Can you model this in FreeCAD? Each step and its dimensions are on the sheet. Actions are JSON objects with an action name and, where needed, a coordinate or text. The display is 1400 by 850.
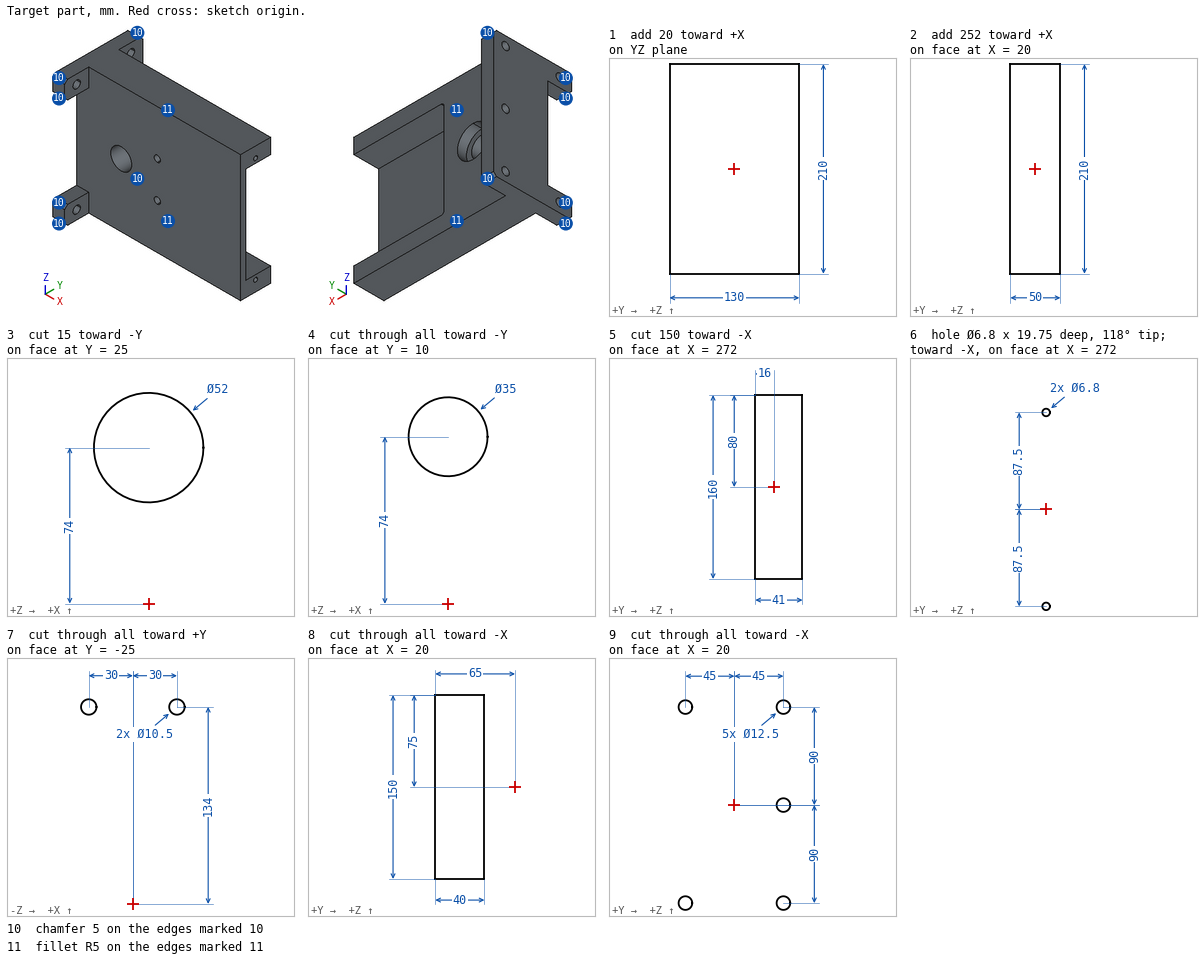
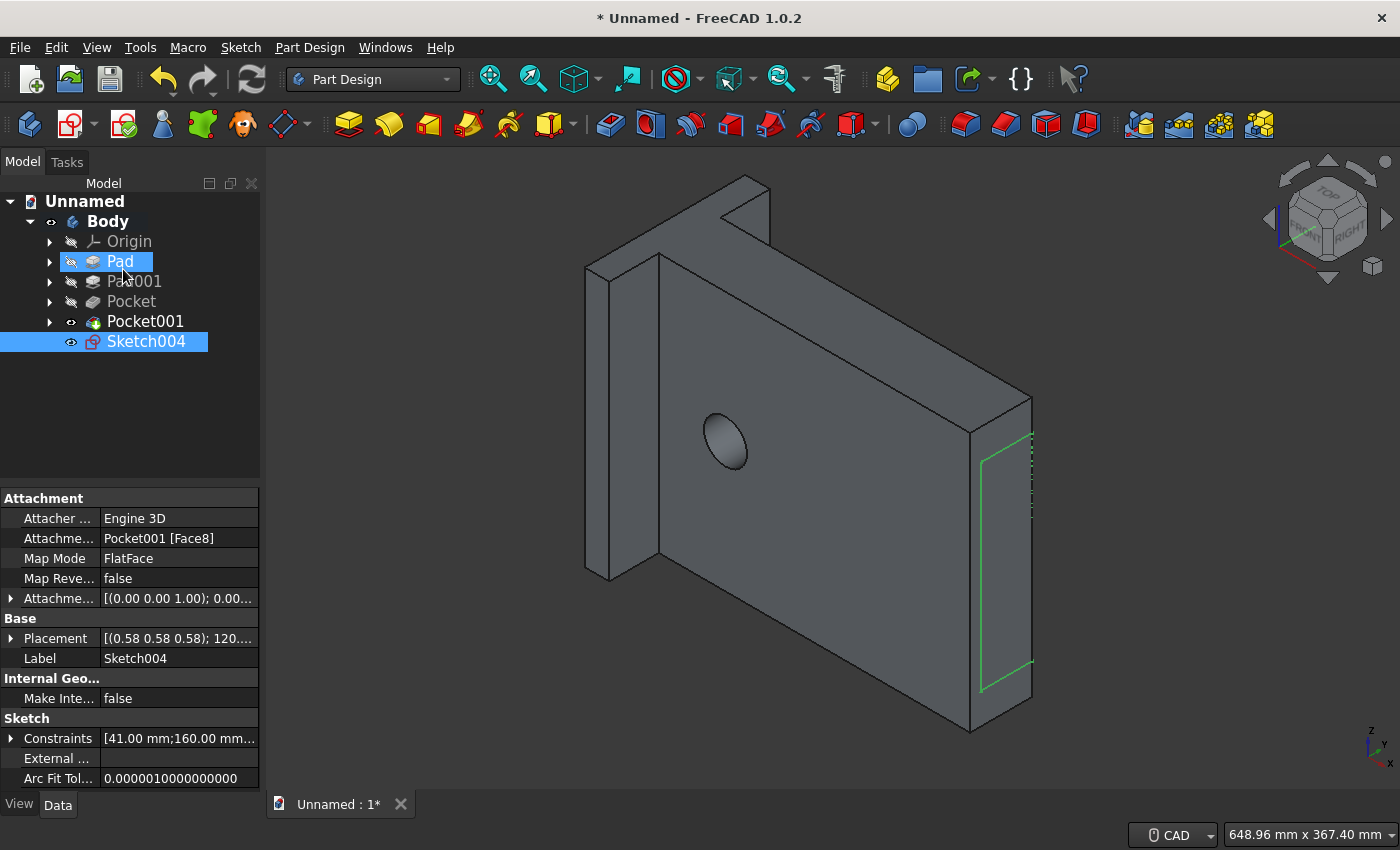
{"action": "left_click", "coordinate": [612, 124]}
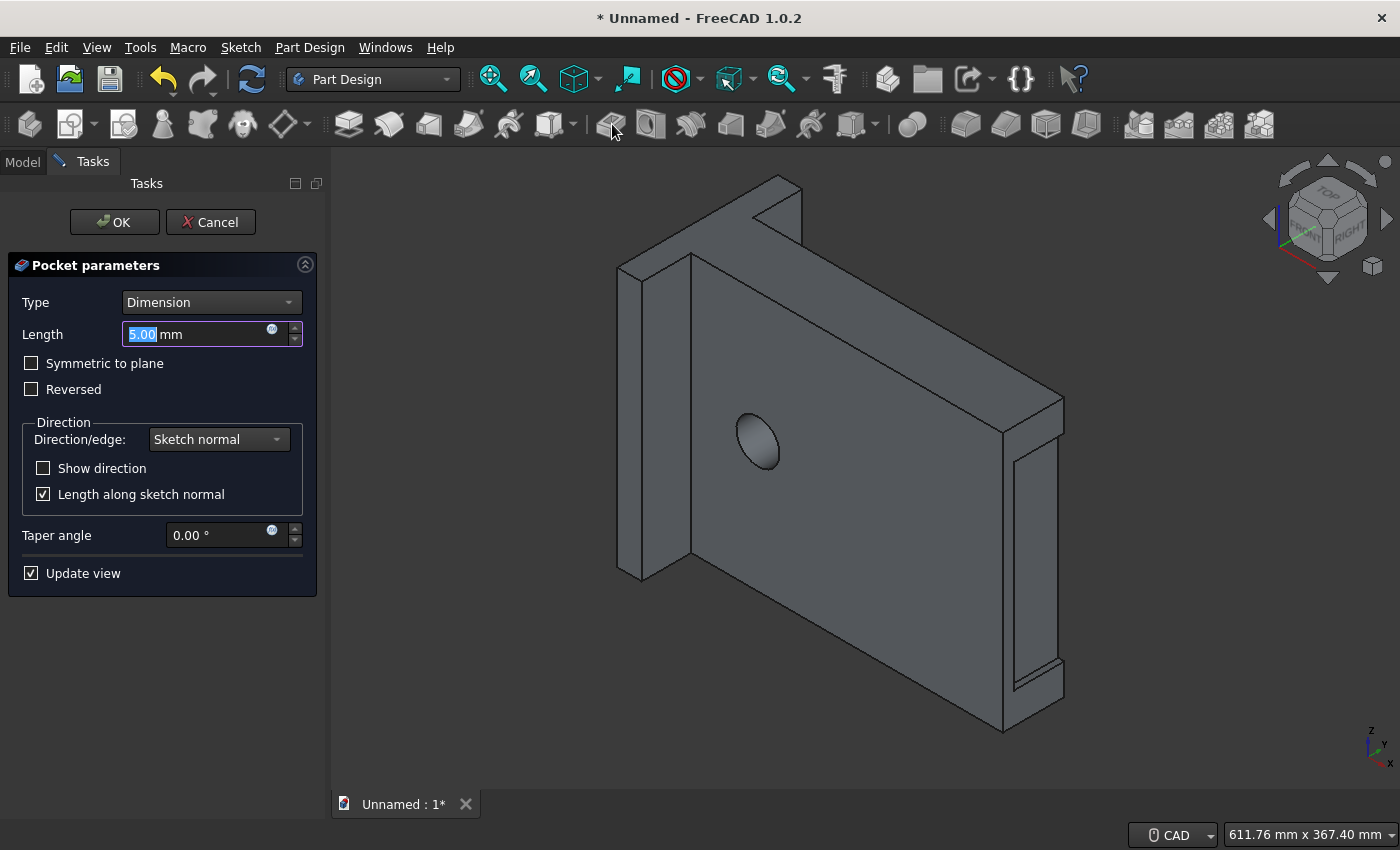
{"action": "type", "text": "150"}
{"action": "key", "text": "Tab"}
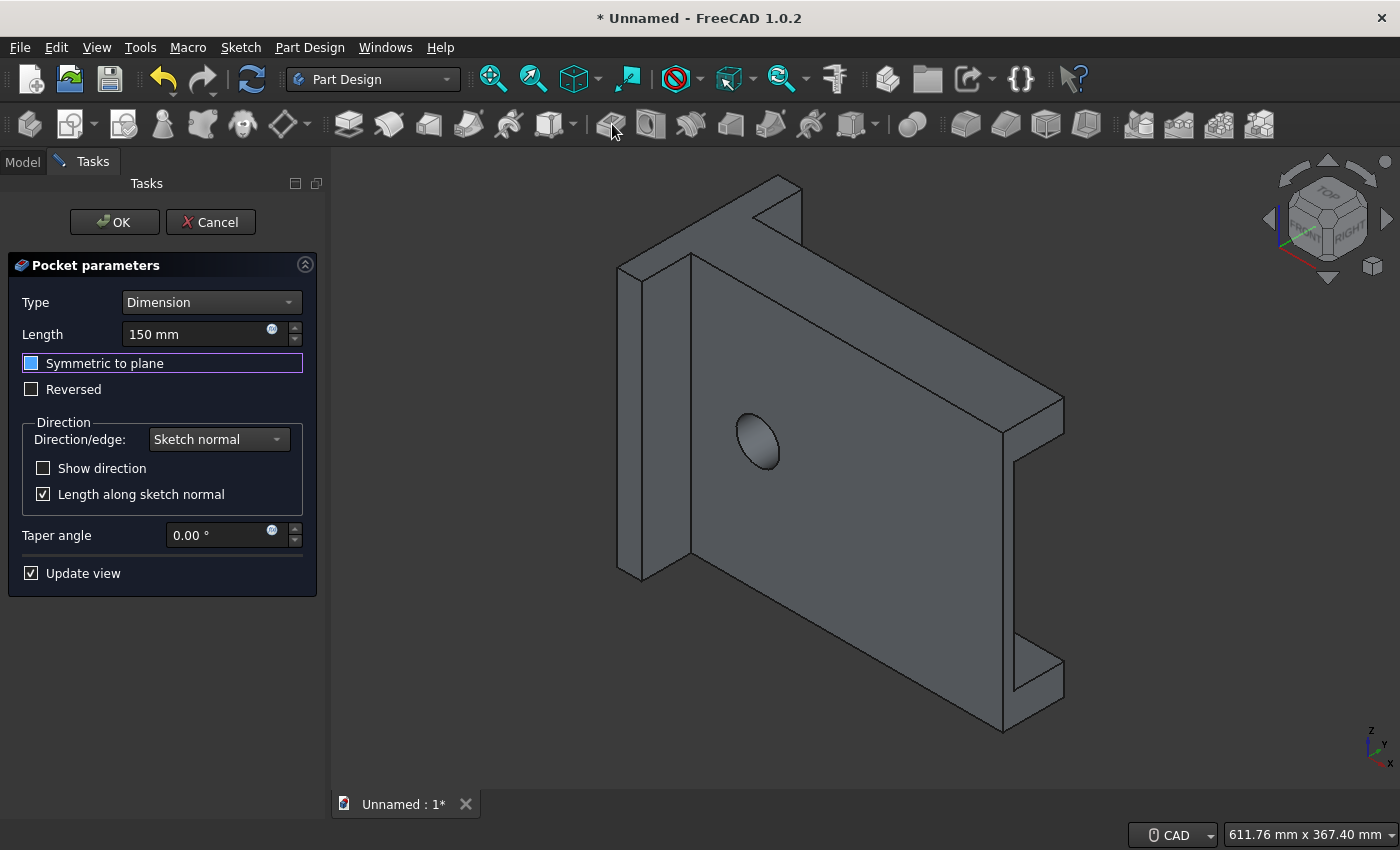
{"action": "left_click", "coordinate": [115, 222]}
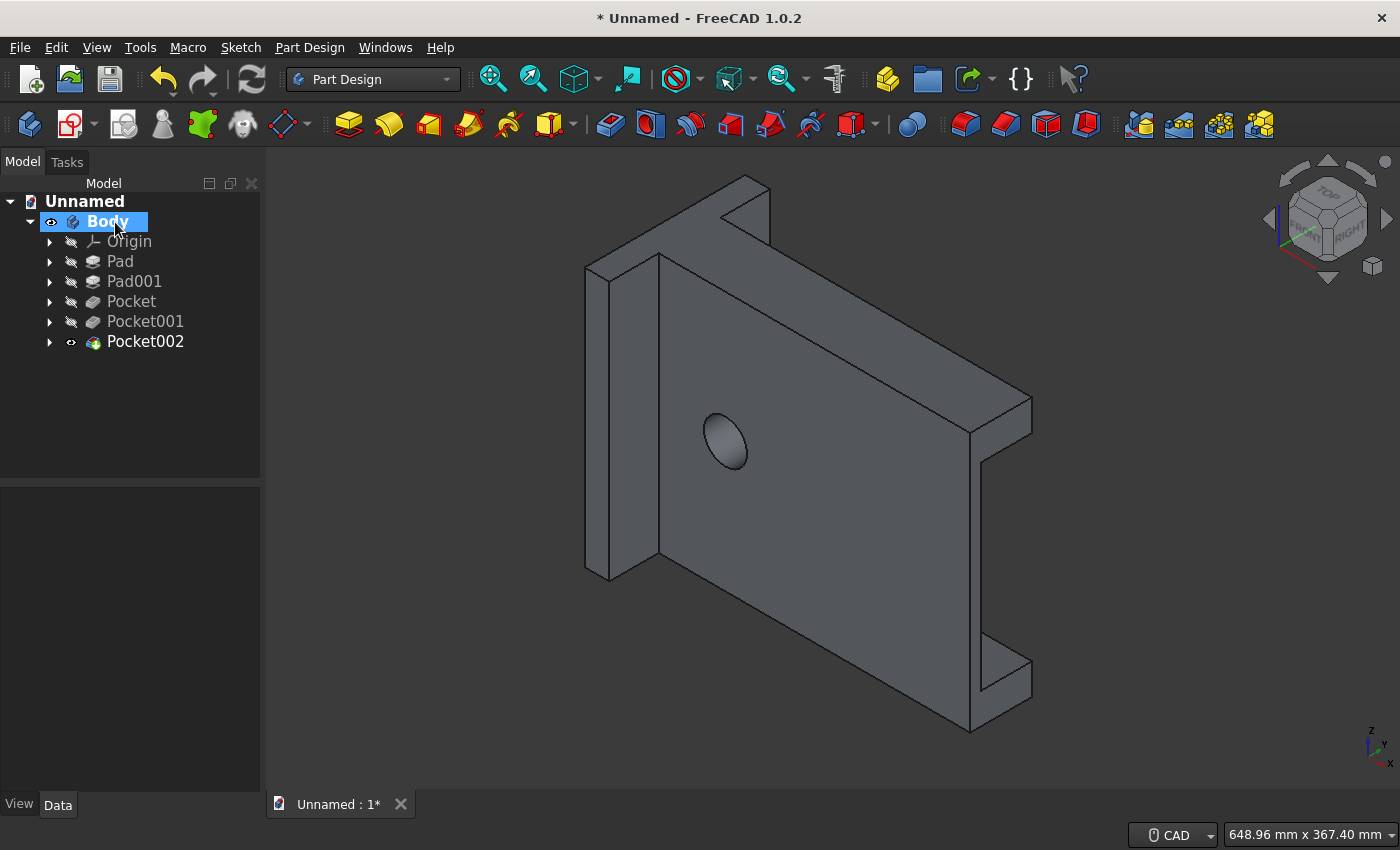
{"action": "left_click", "coordinate": [1019, 682]}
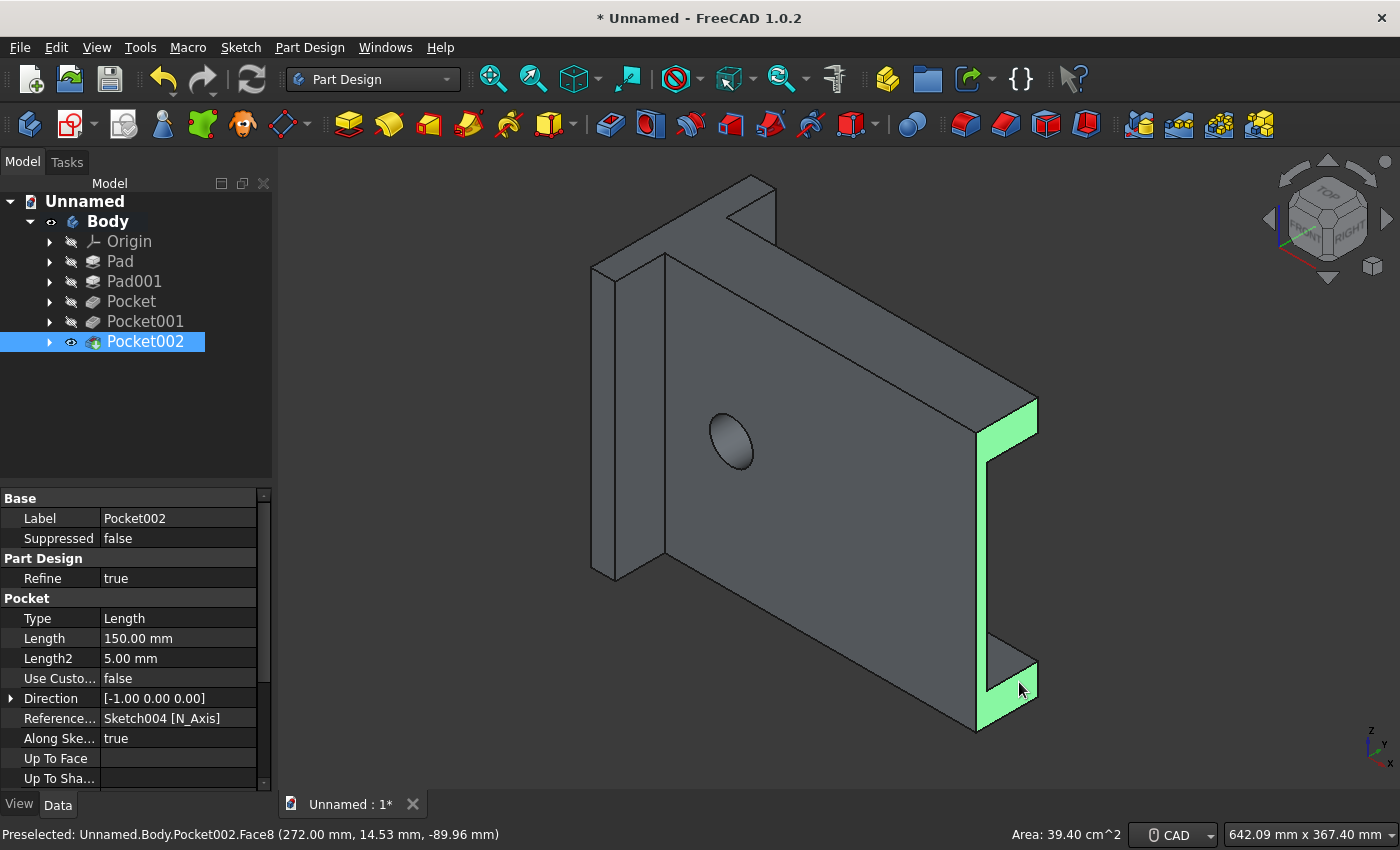
{"action": "left_click", "coordinate": [70, 124]}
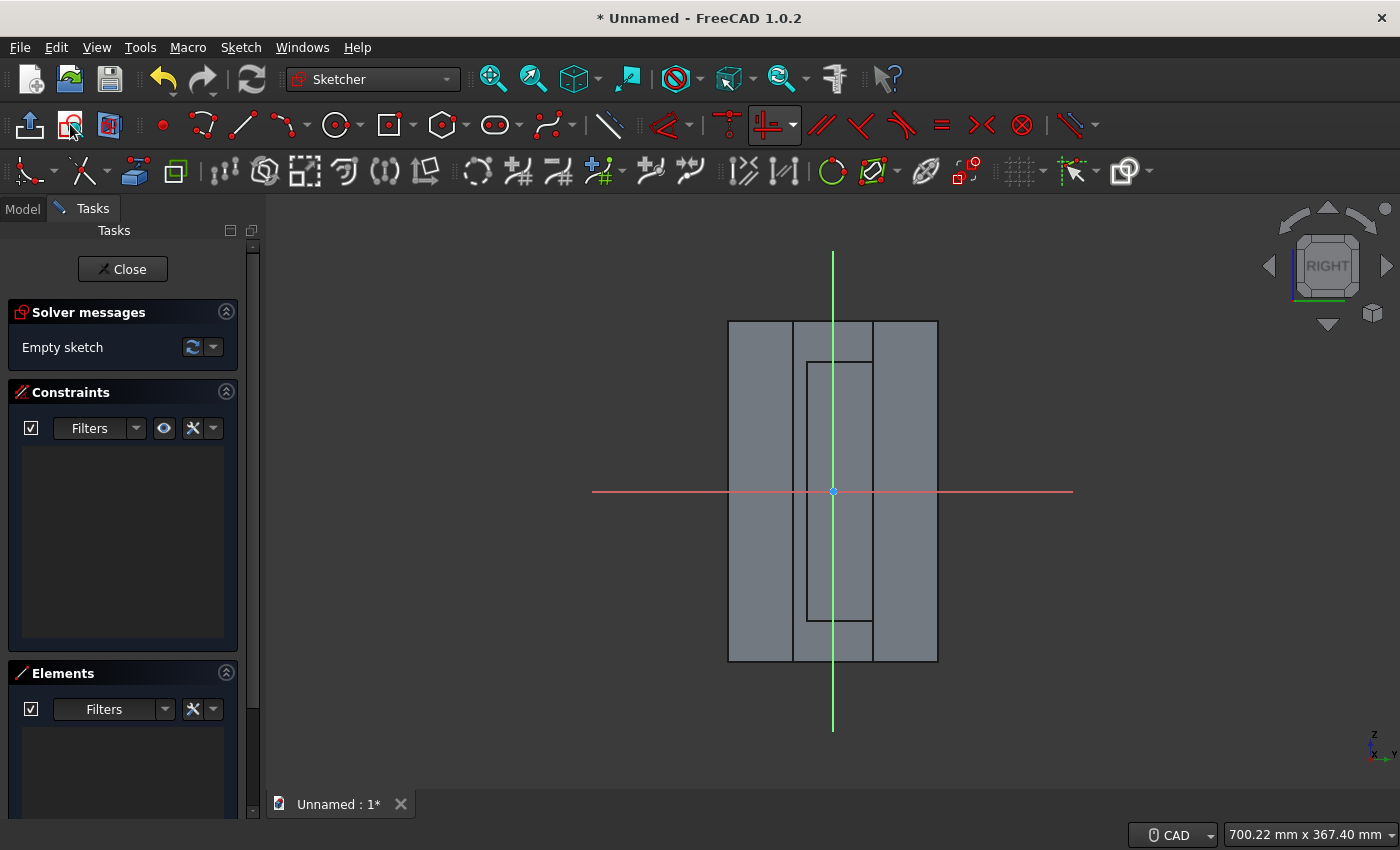
{"action": "left_click", "coordinate": [336, 126]}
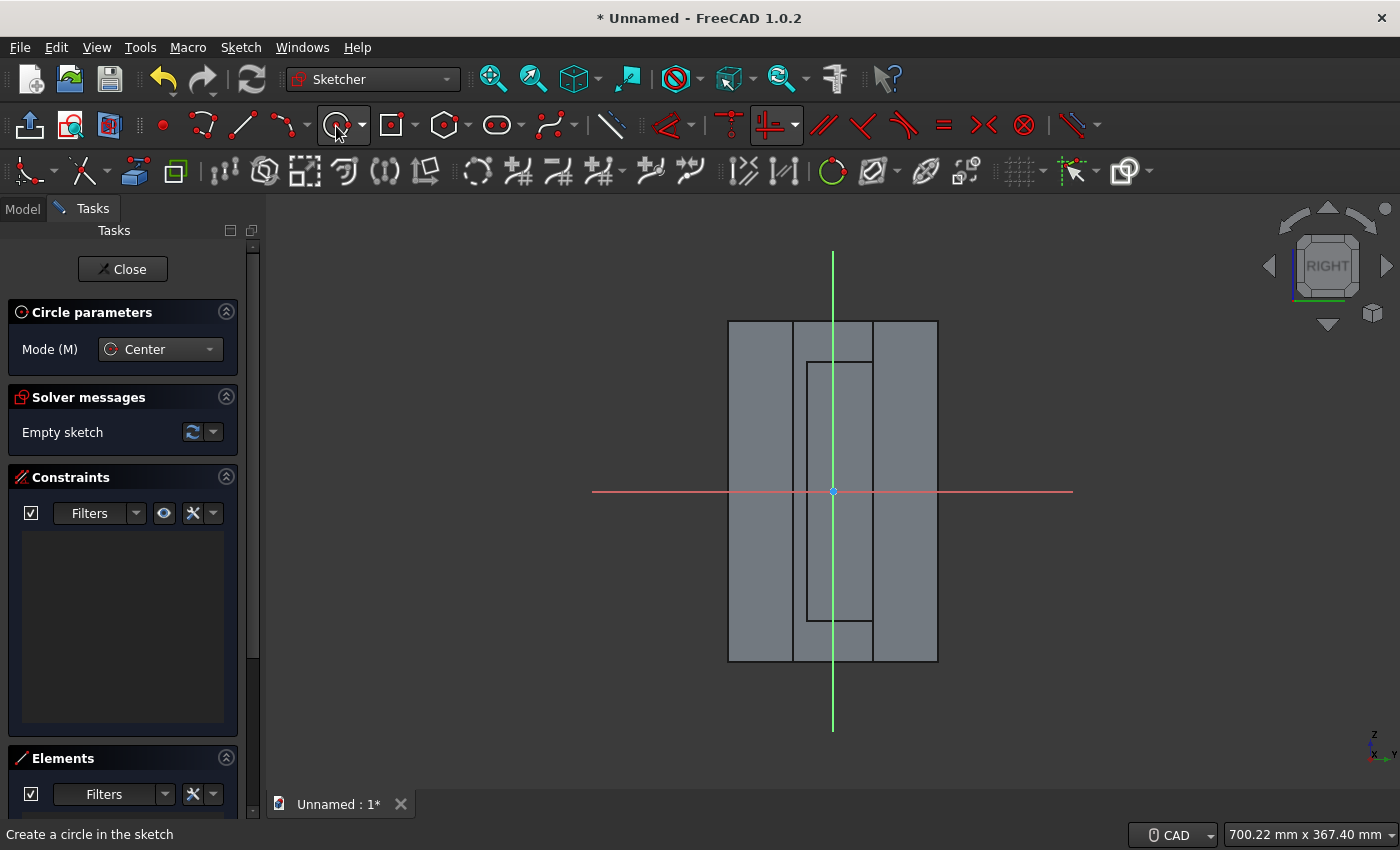
{"action": "scroll", "coordinate": [833, 350], "scroll_direction": "up", "scroll_amount": 8}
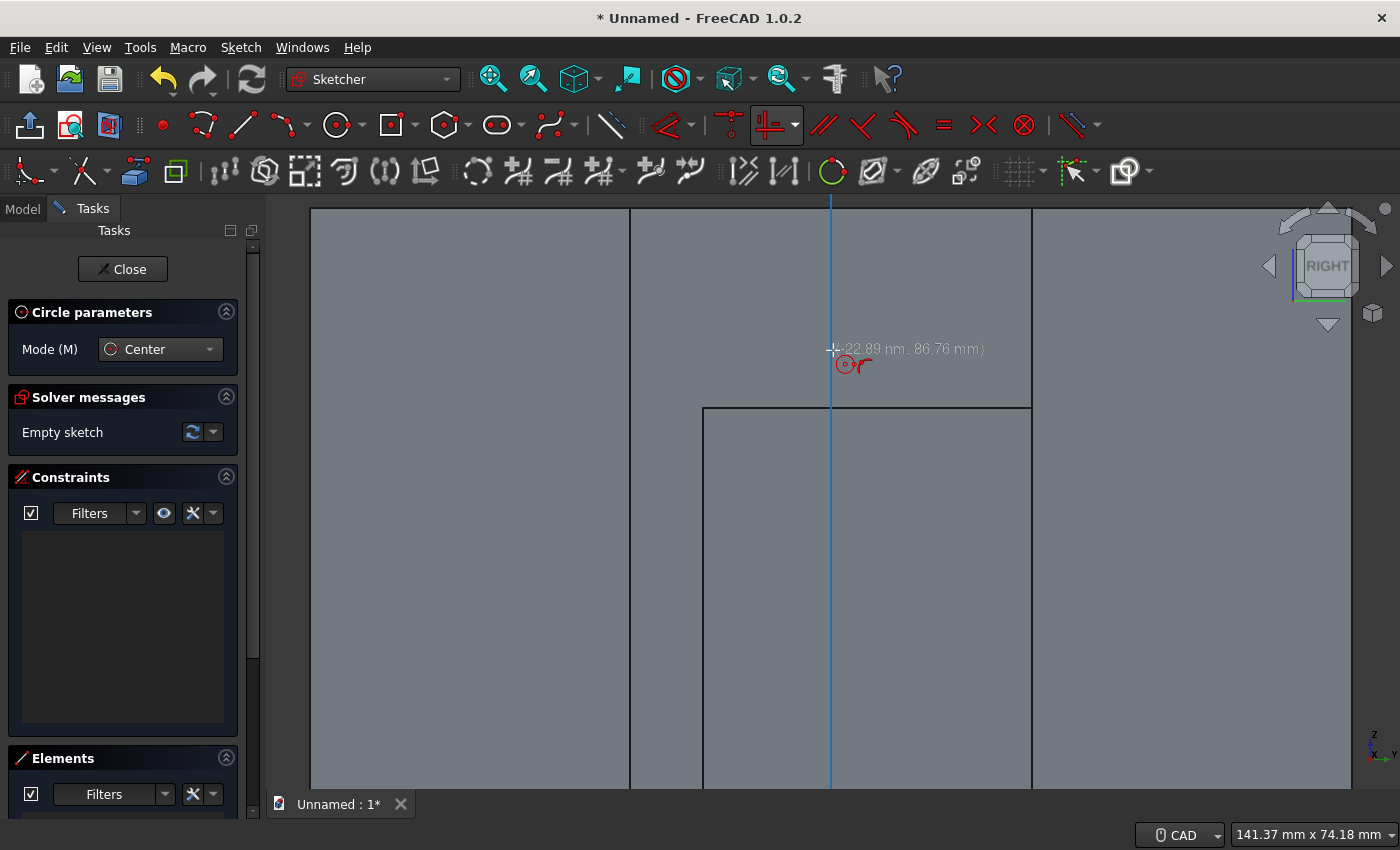
{"action": "scroll", "coordinate": [743, 309], "scroll_direction": "down", "scroll_amount": 7}